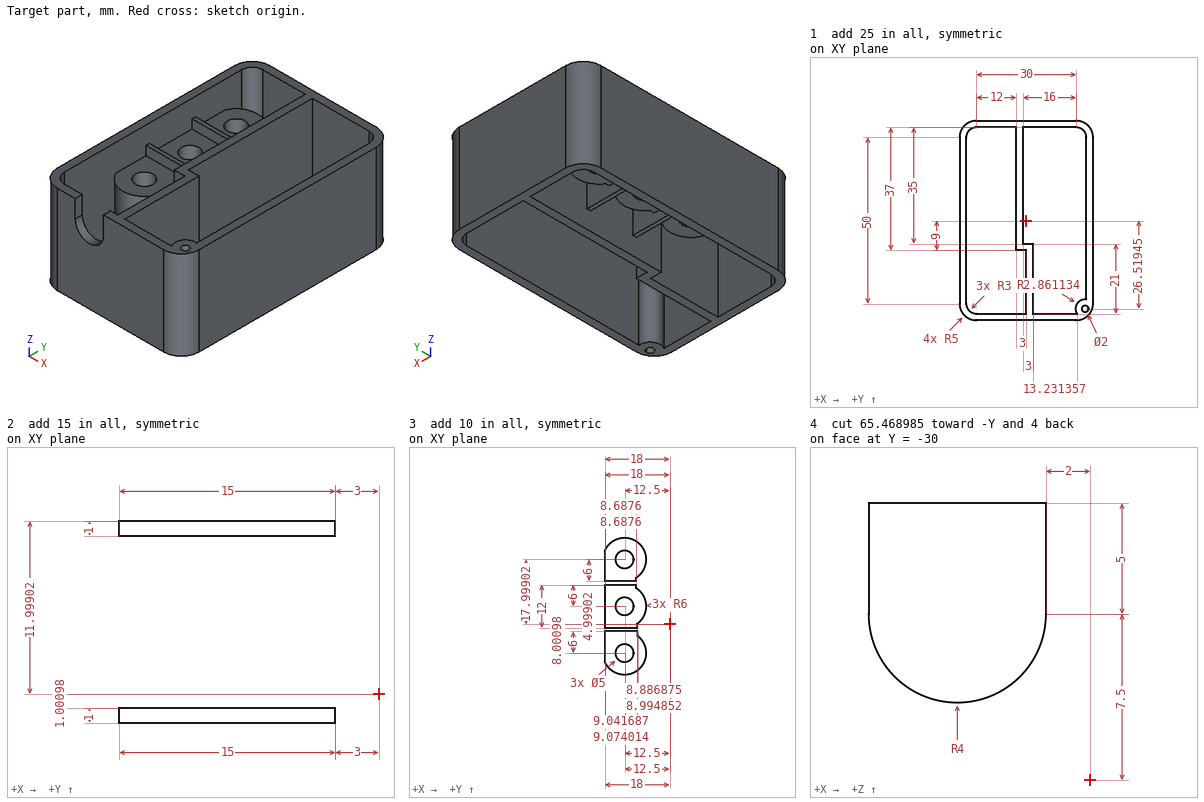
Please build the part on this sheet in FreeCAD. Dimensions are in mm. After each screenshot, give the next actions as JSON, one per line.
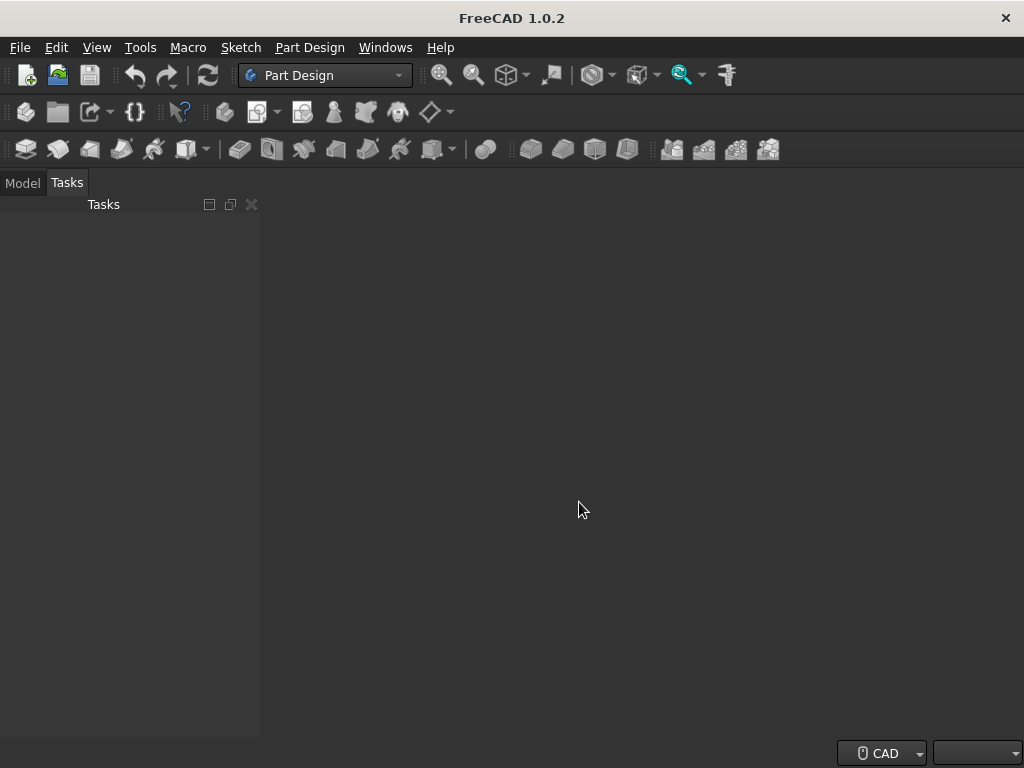
{"action": "left_click", "coordinate": [26, 76]}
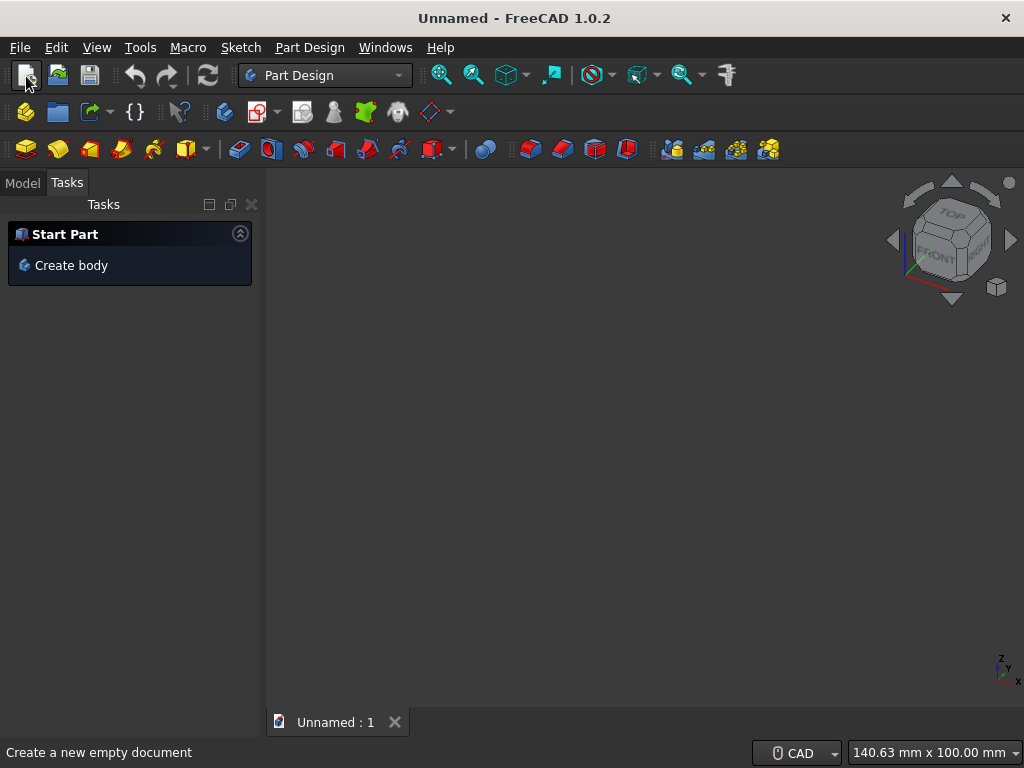
{"action": "left_click", "coordinate": [258, 112]}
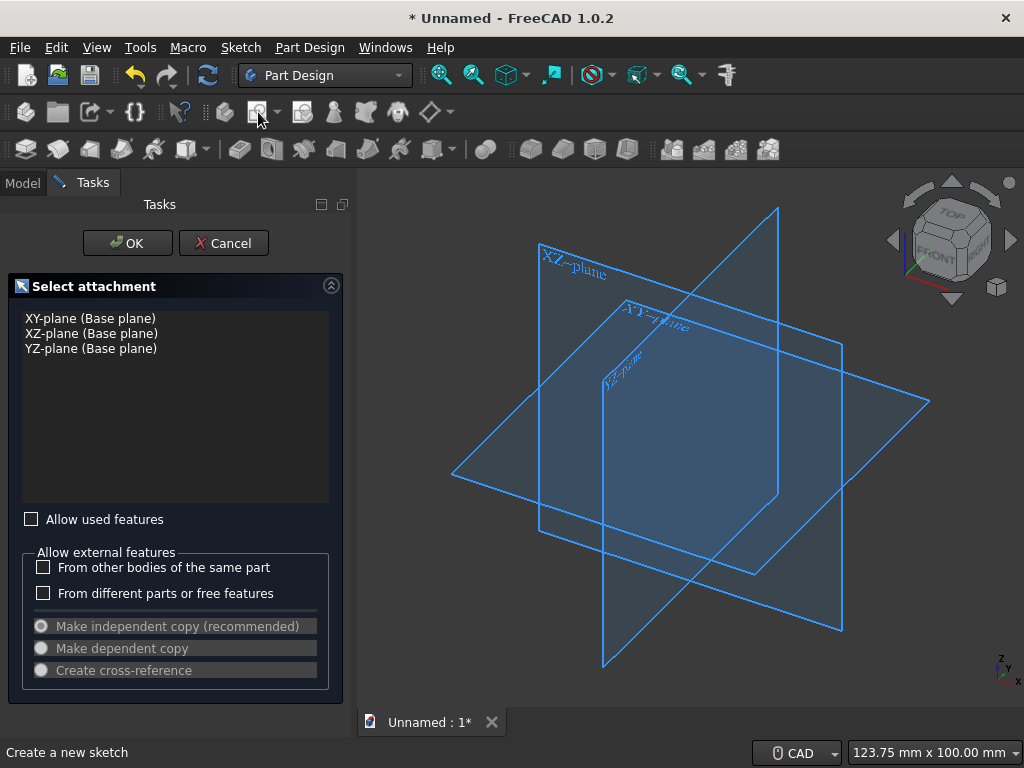
{"action": "left_click", "coordinate": [82, 318]}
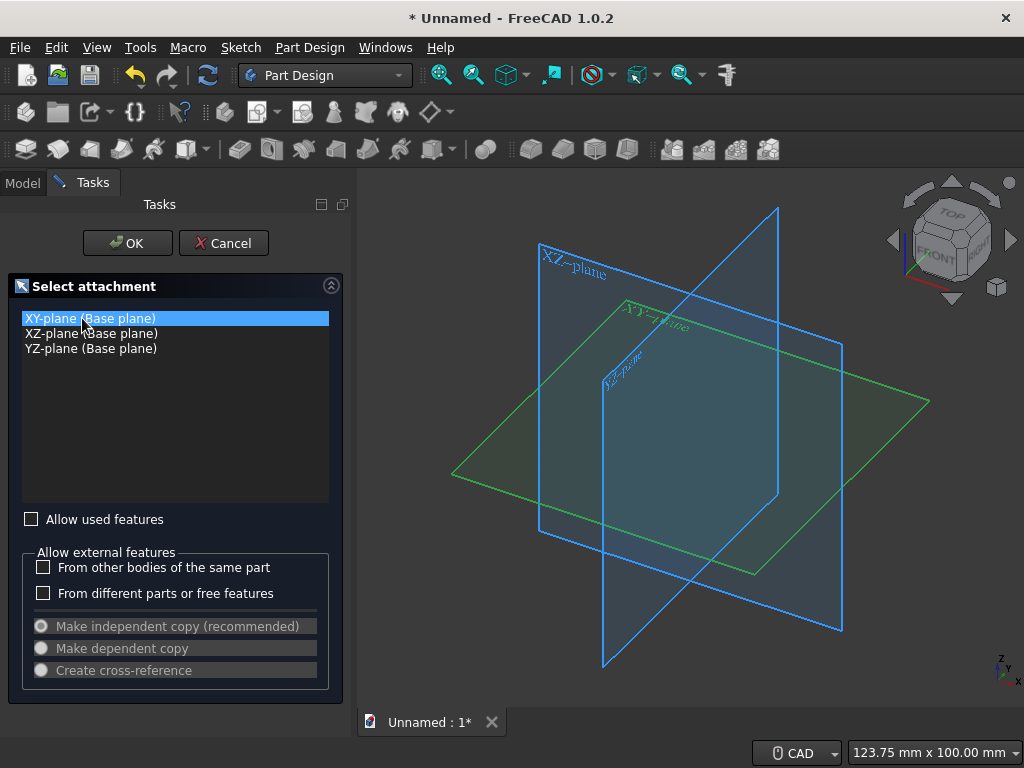
{"action": "left_click", "coordinate": [128, 243]}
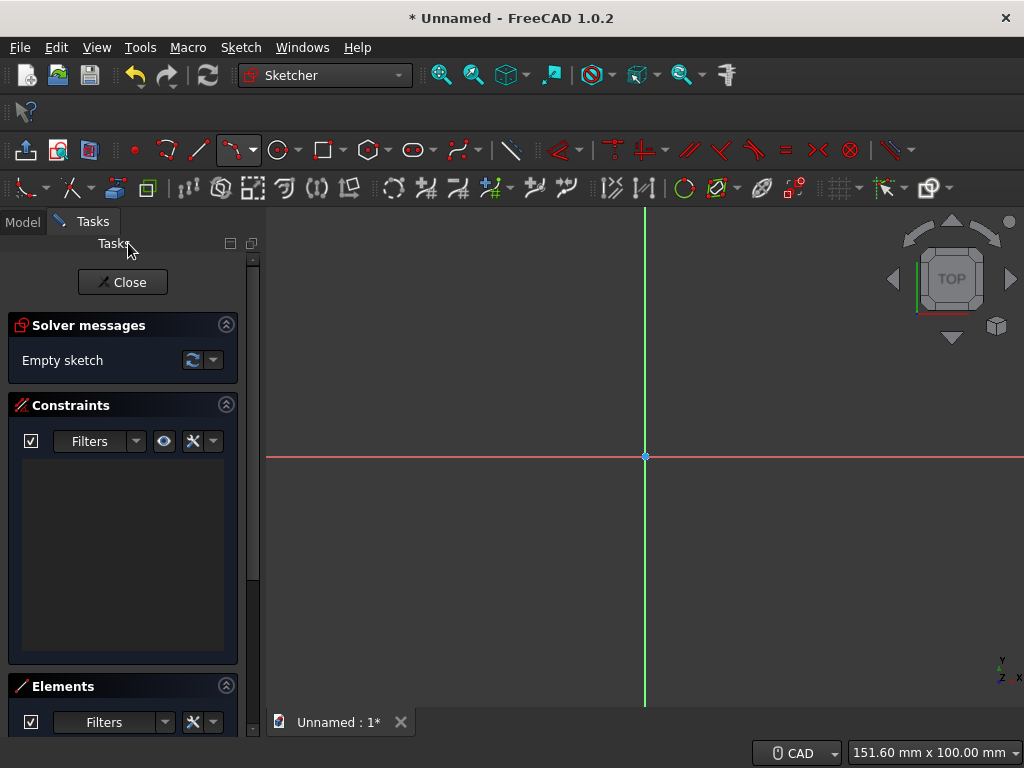
{"action": "left_click", "coordinate": [200, 150]}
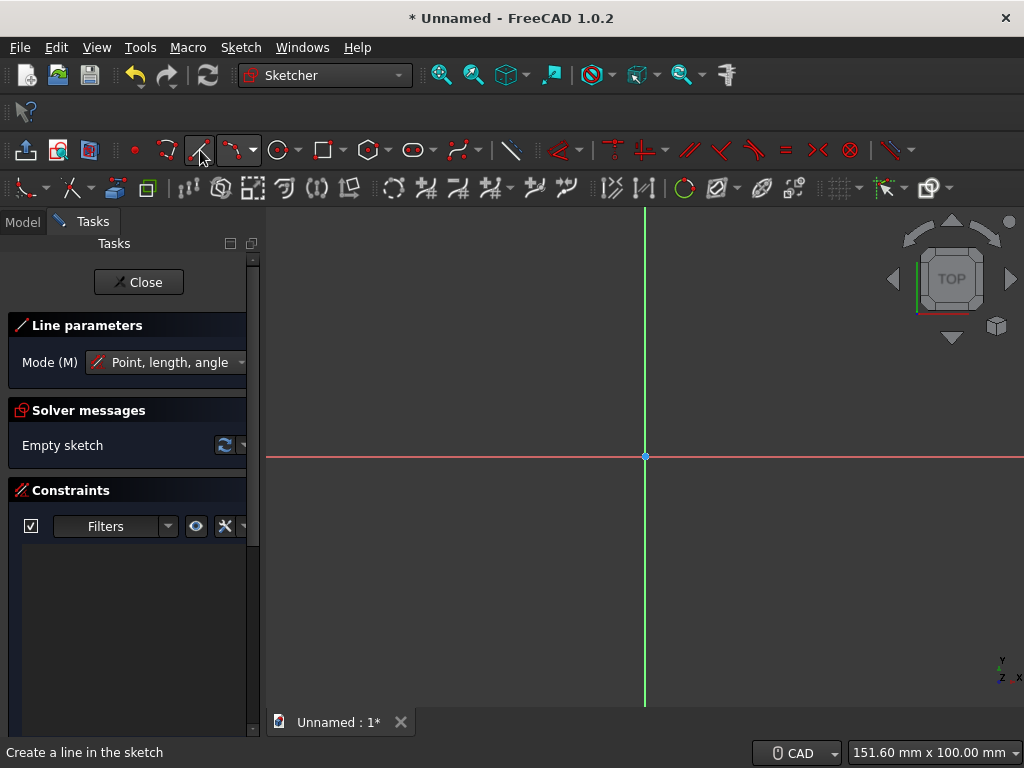
{"action": "left_click", "coordinate": [720, 307]}
{"action": "left_click", "coordinate": [570, 307]}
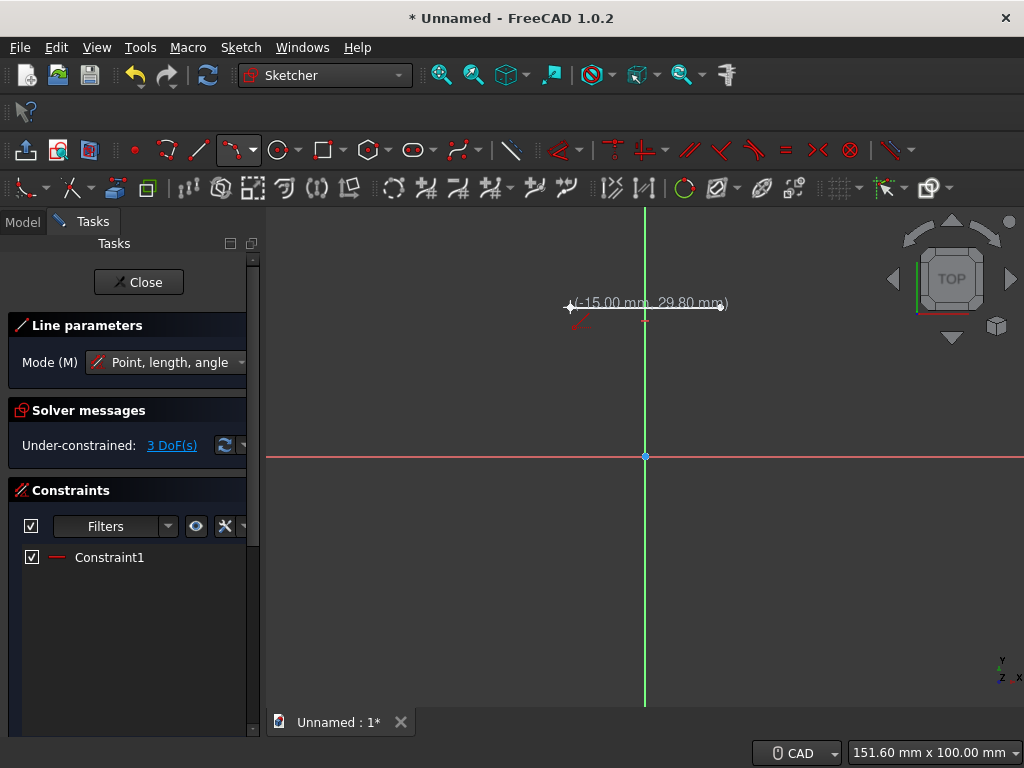
{"action": "left_click", "coordinate": [545, 332]}
{"action": "left_click", "coordinate": [545, 582]}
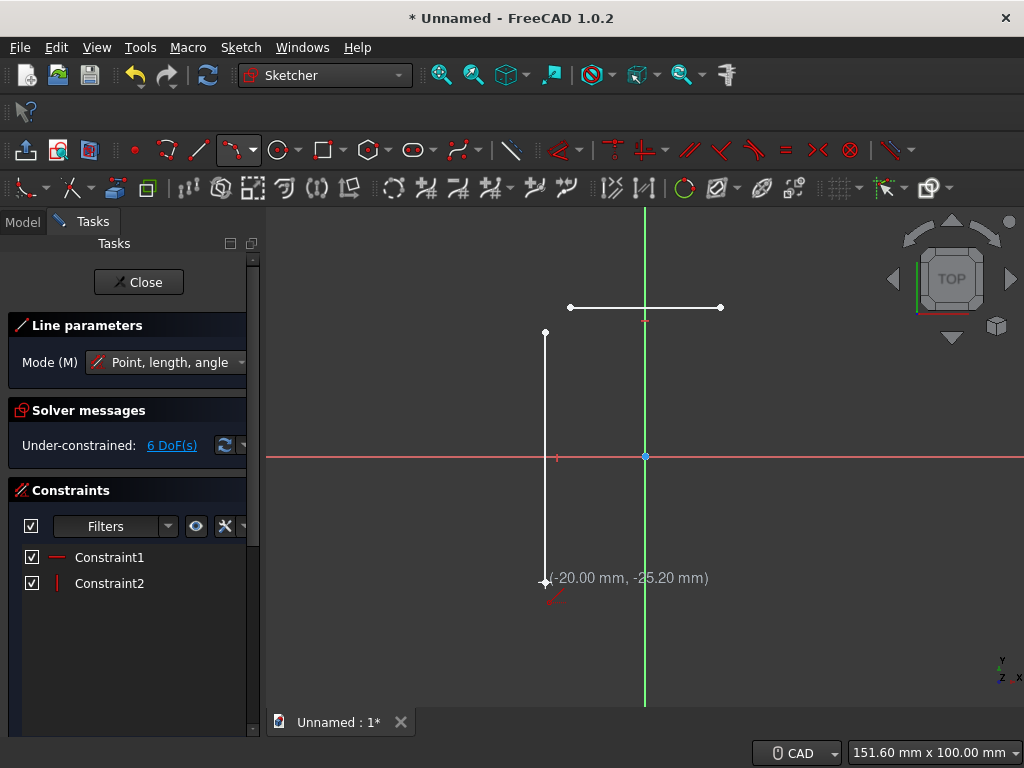
{"action": "left_click", "coordinate": [570, 607]}
{"action": "left_click", "coordinate": [720, 607]}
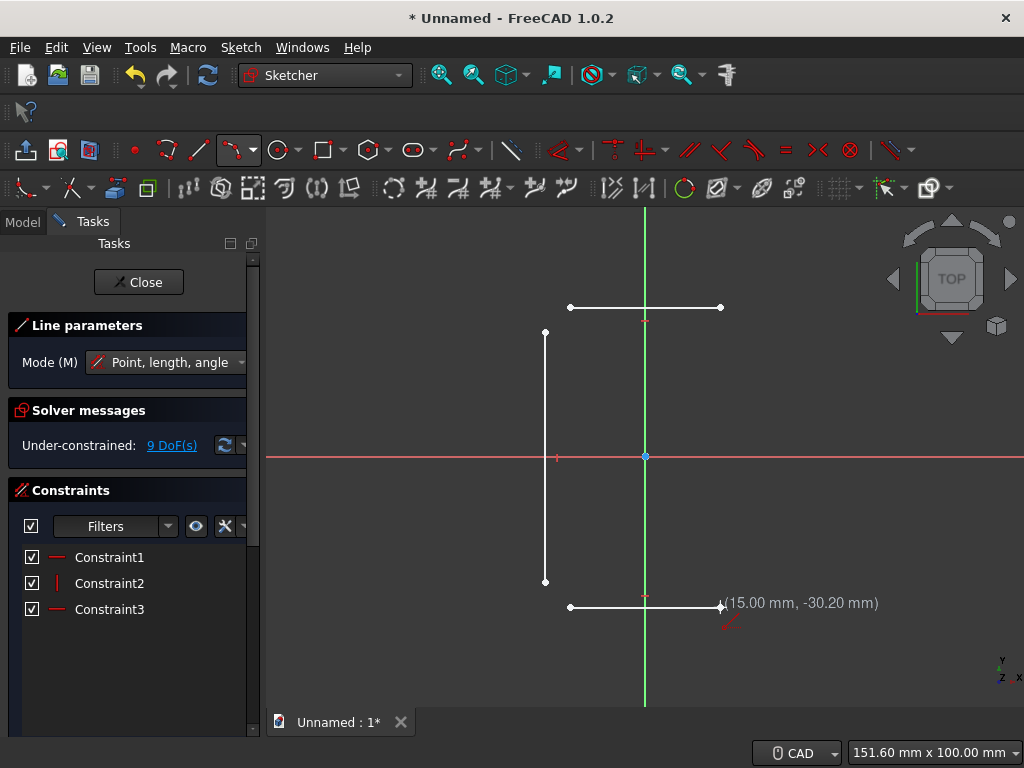
{"action": "left_click", "coordinate": [745, 582]}
{"action": "left_click", "coordinate": [745, 332]}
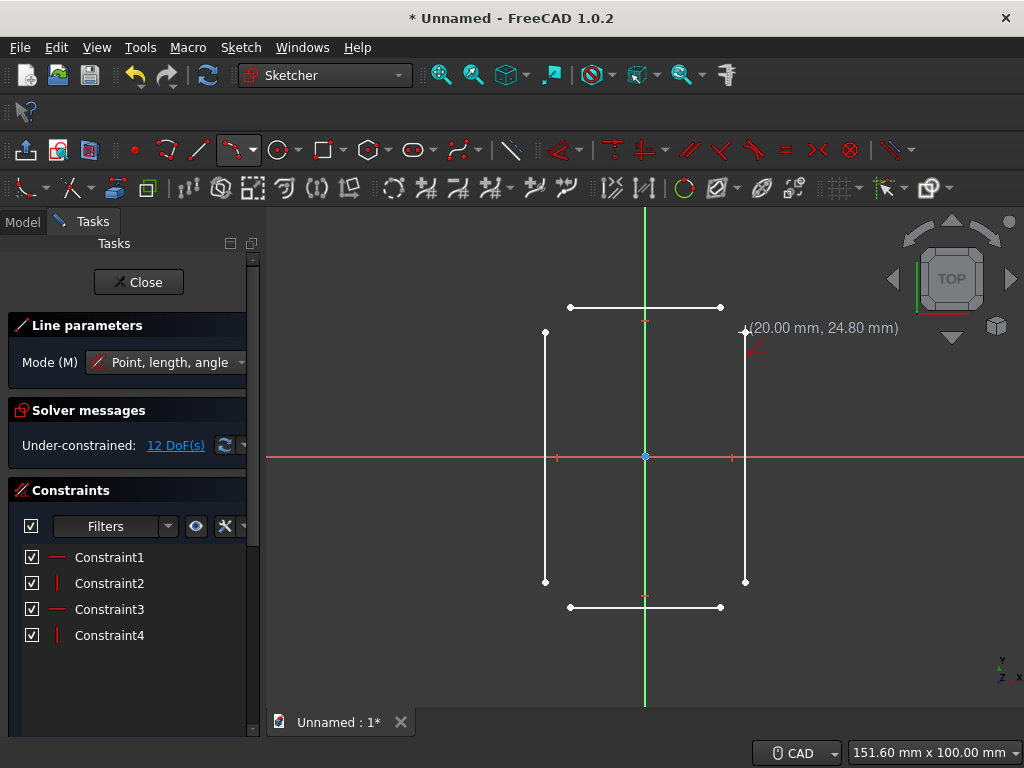
{"action": "left_click", "coordinate": [232, 150]}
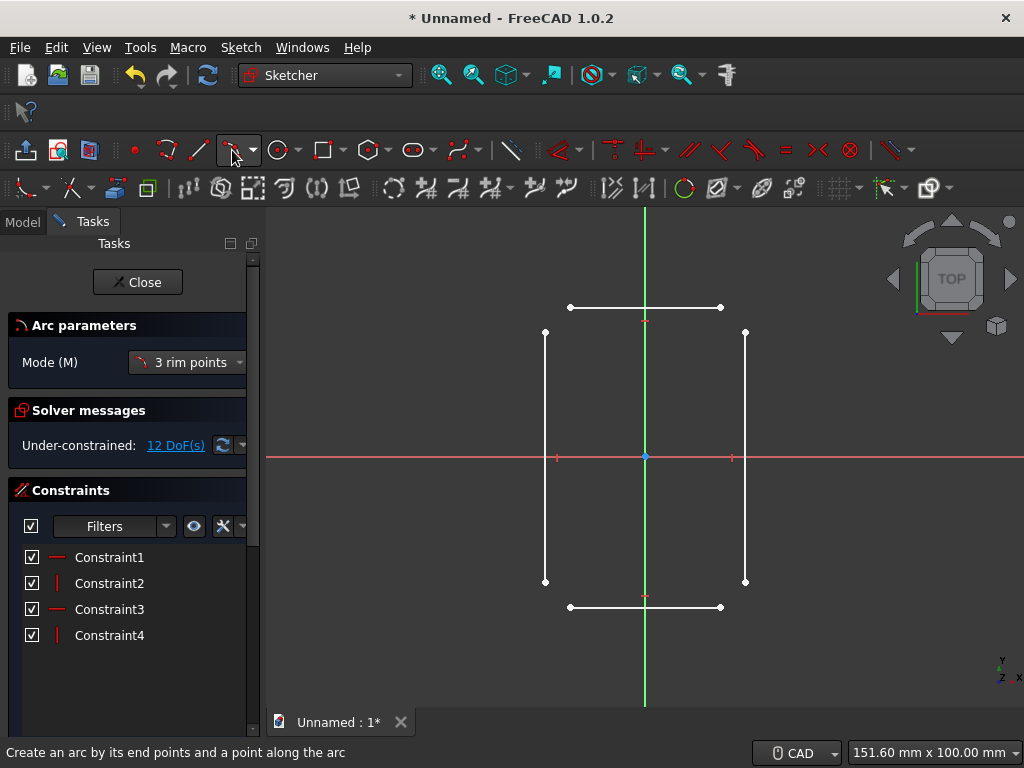
{"action": "left_click", "coordinate": [570, 308]}
{"action": "left_click", "coordinate": [545, 333]}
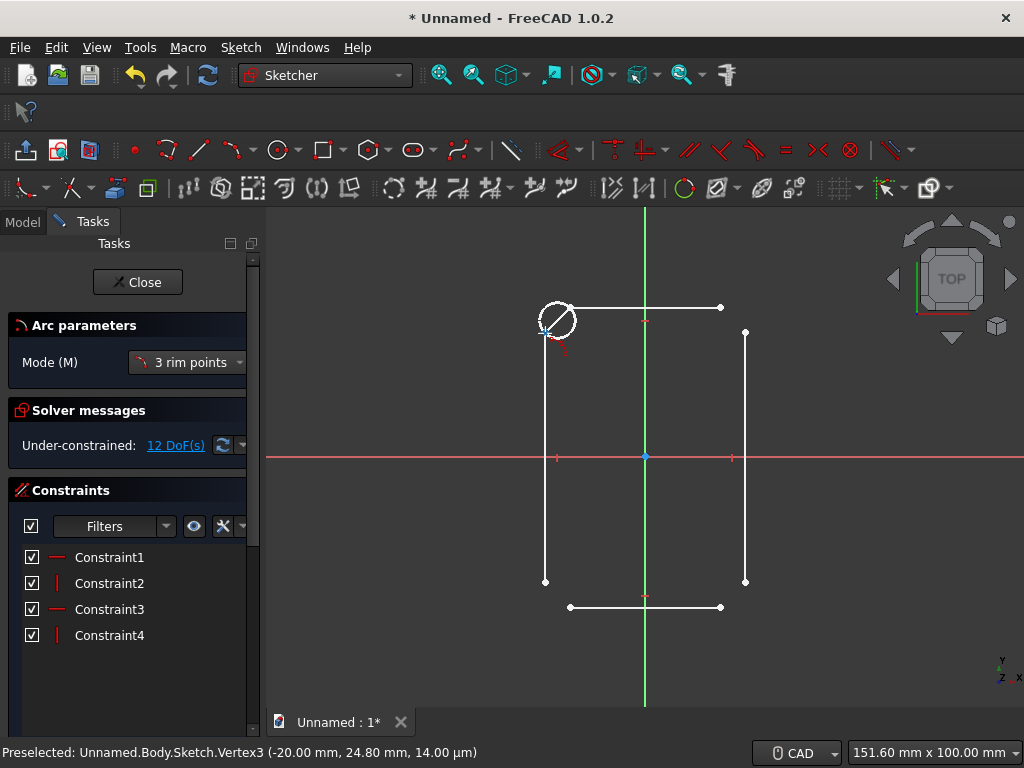
{"action": "scroll", "coordinate": [552, 314], "scroll_direction": "up", "scroll_amount": 4}